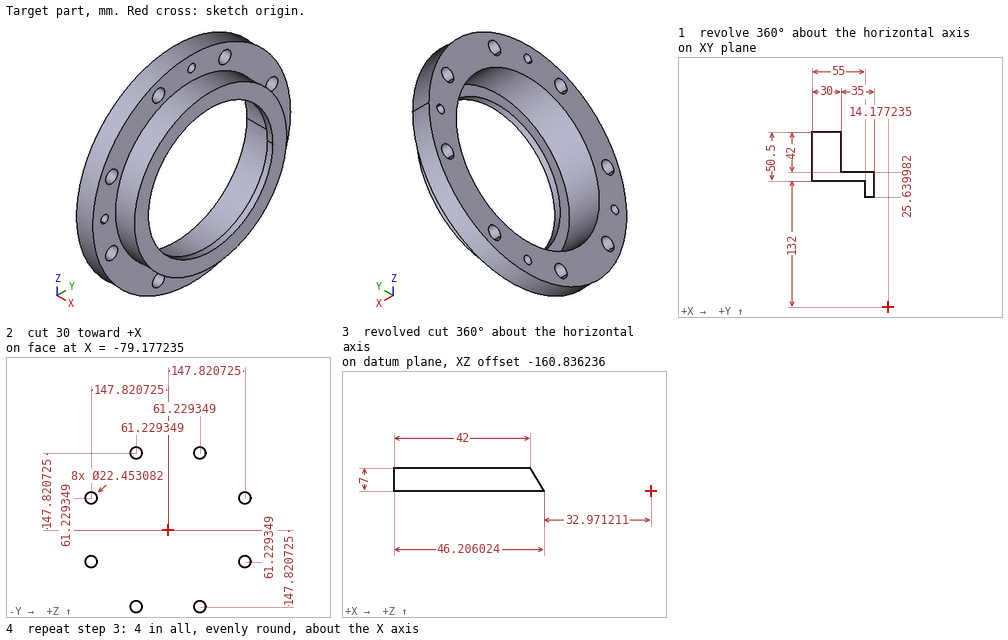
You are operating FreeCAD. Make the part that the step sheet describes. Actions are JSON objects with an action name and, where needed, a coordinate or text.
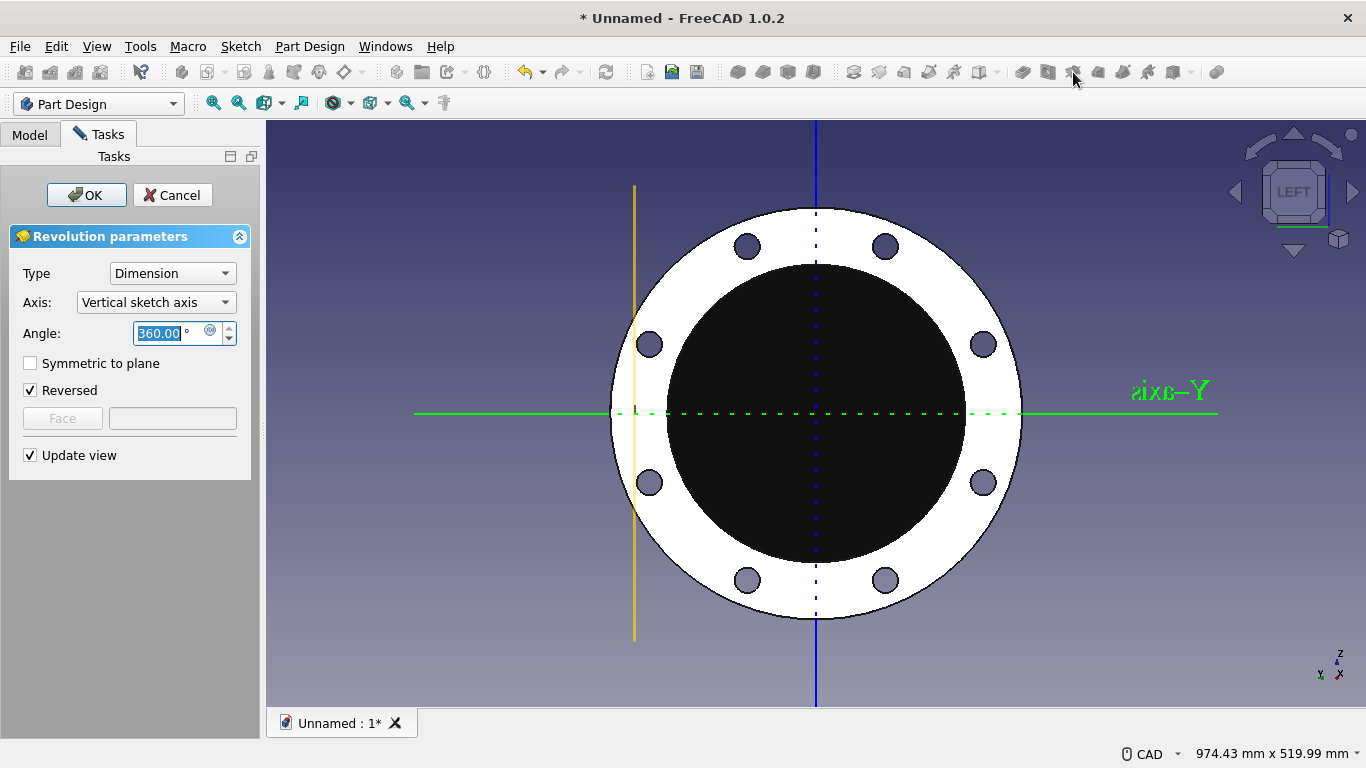
{"action": "left_click", "coordinate": [157, 302]}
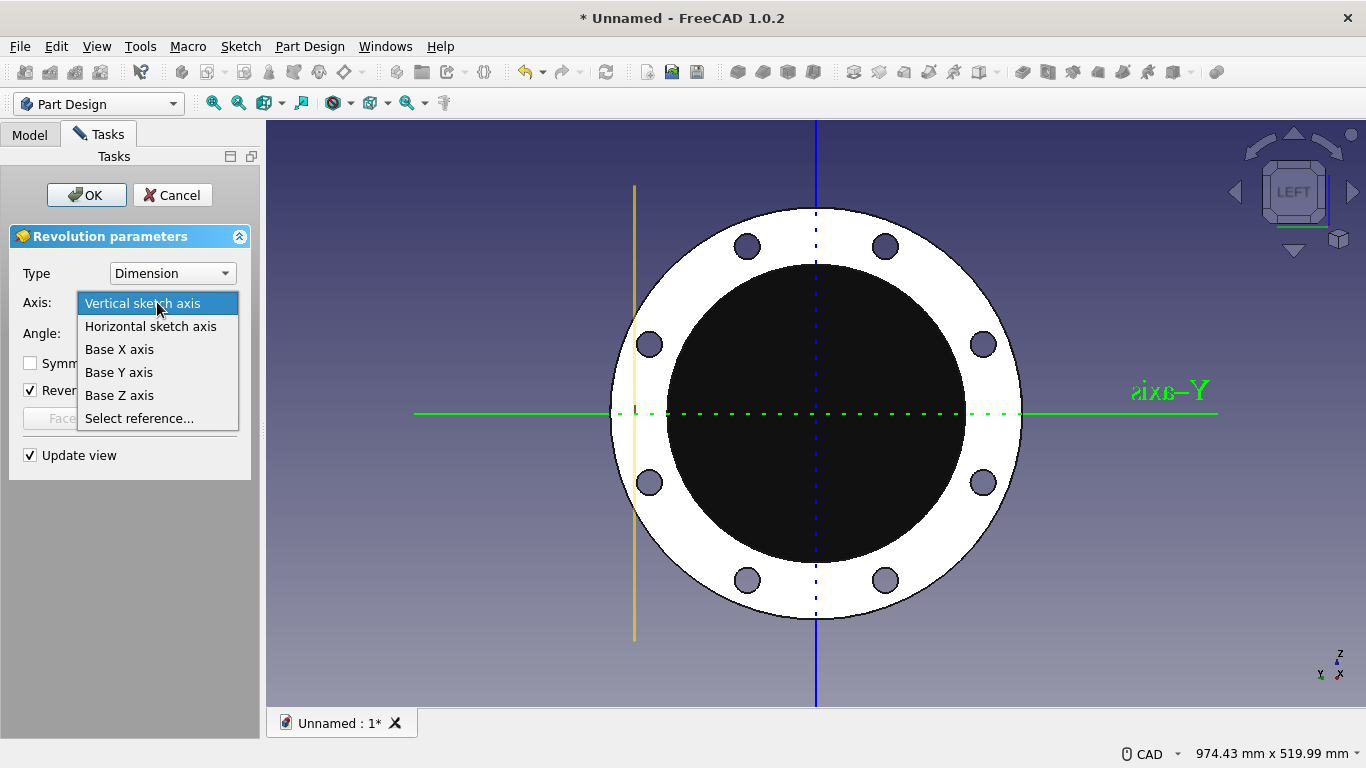
{"action": "left_click", "coordinate": [156, 326]}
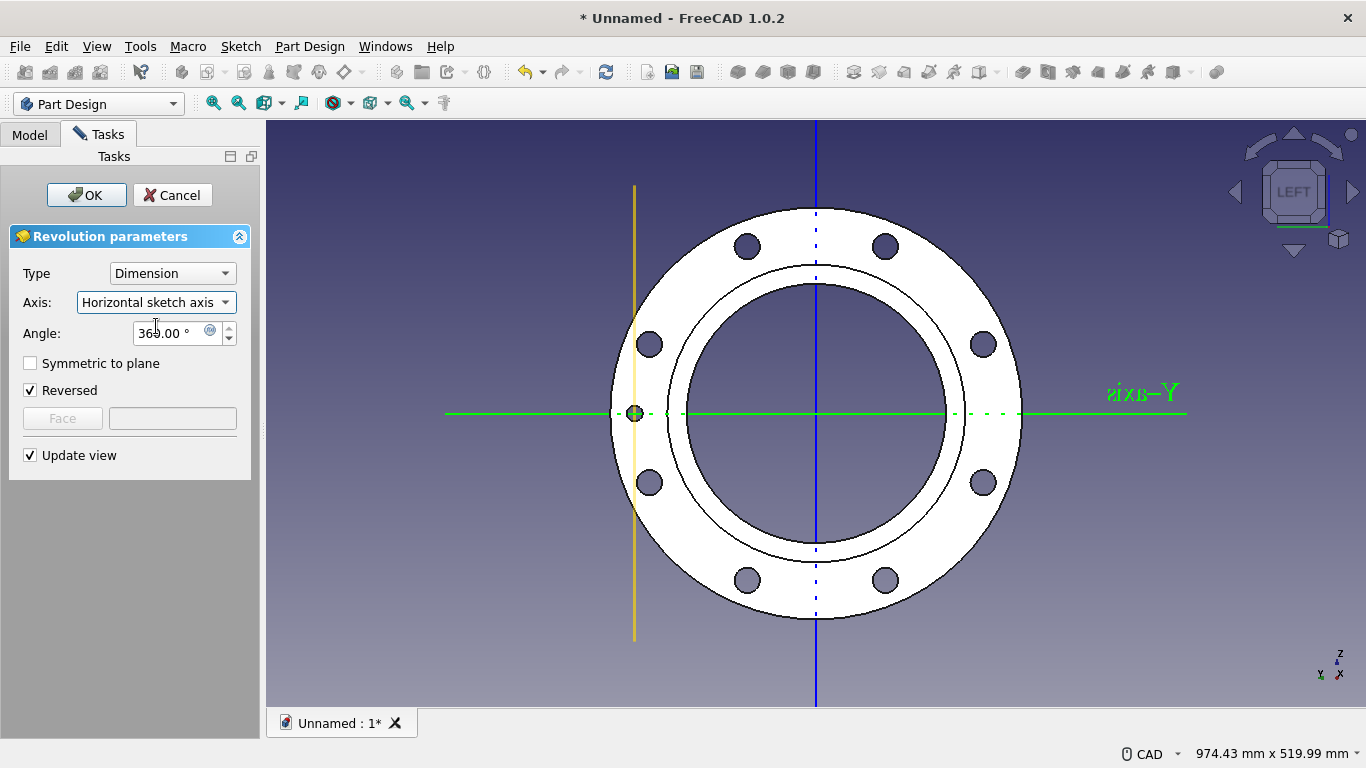
{"action": "left_click", "coordinate": [87, 195]}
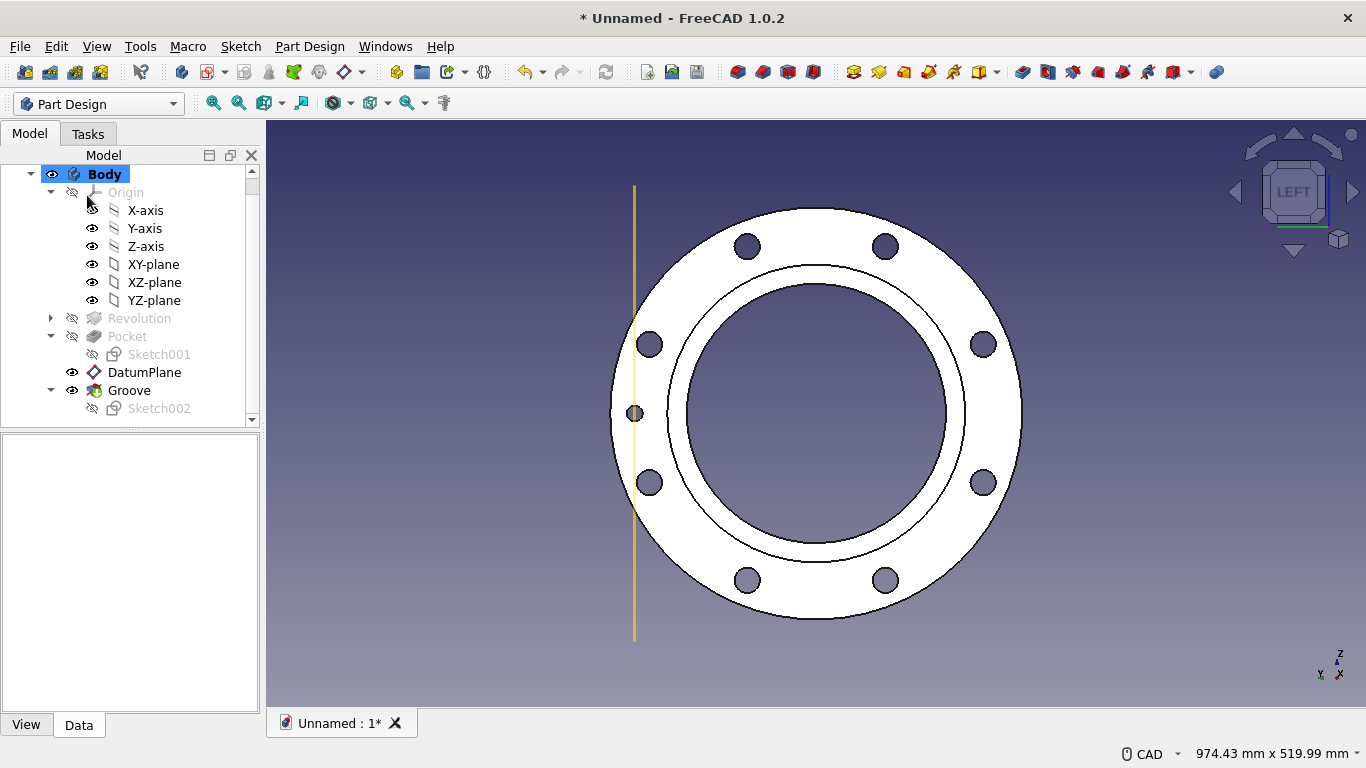
{"action": "left_click", "coordinate": [117, 372]}
{"action": "key", "text": "space"}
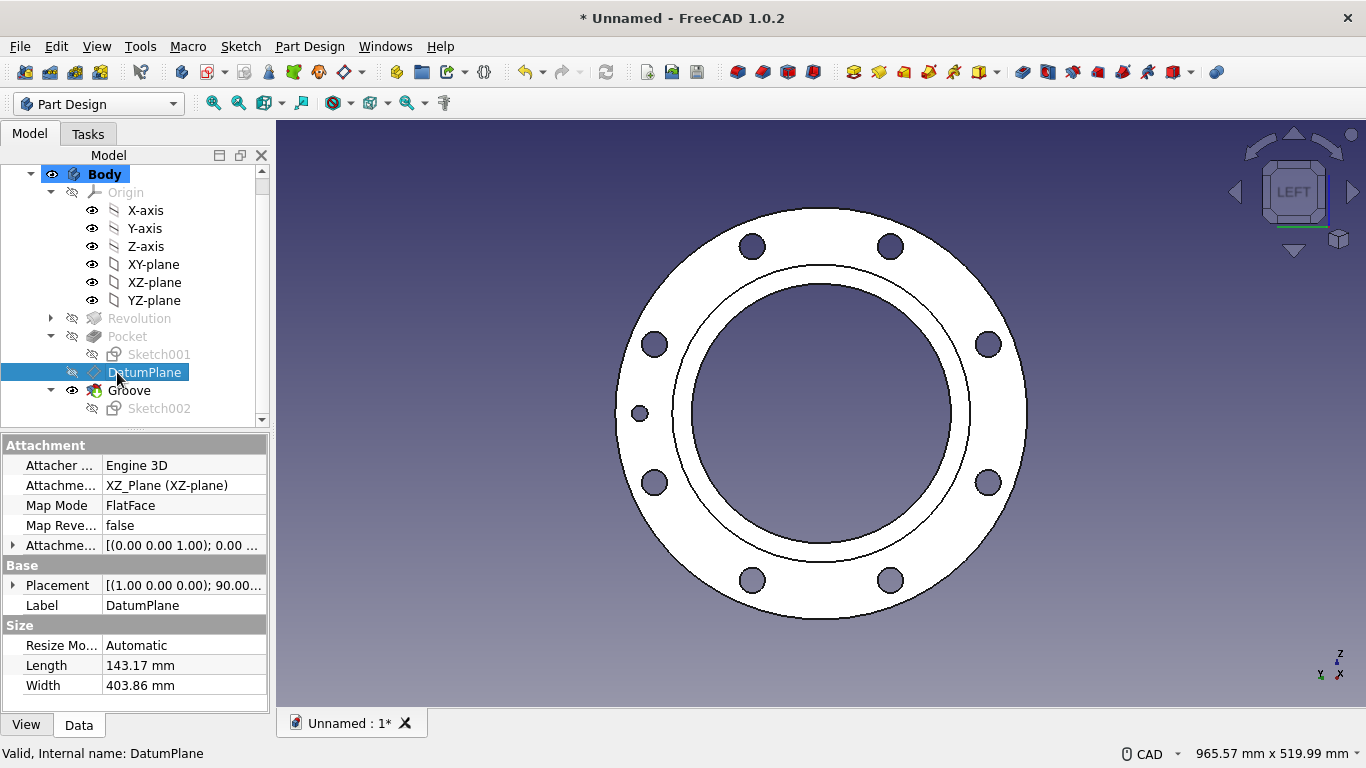
{"action": "left_click", "coordinate": [117, 390]}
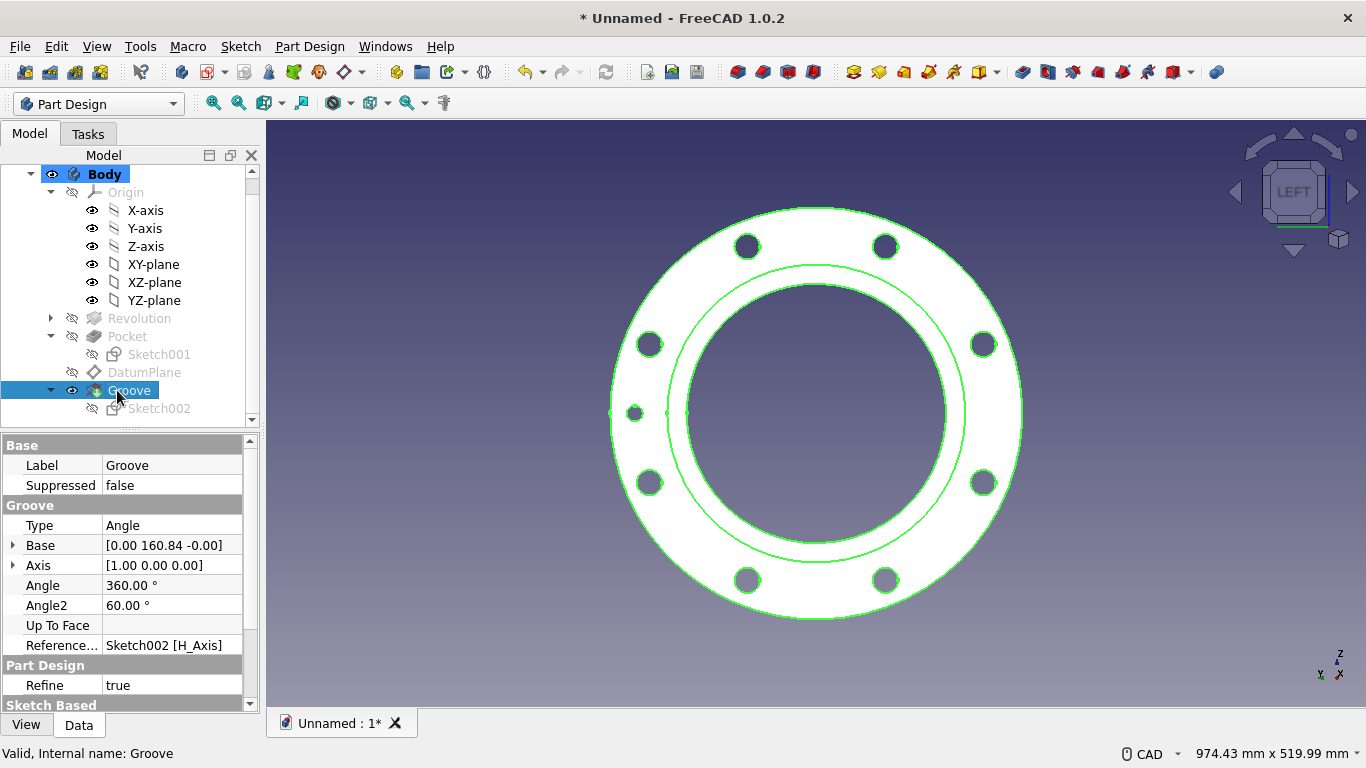
{"action": "left_click", "coordinate": [75, 72]}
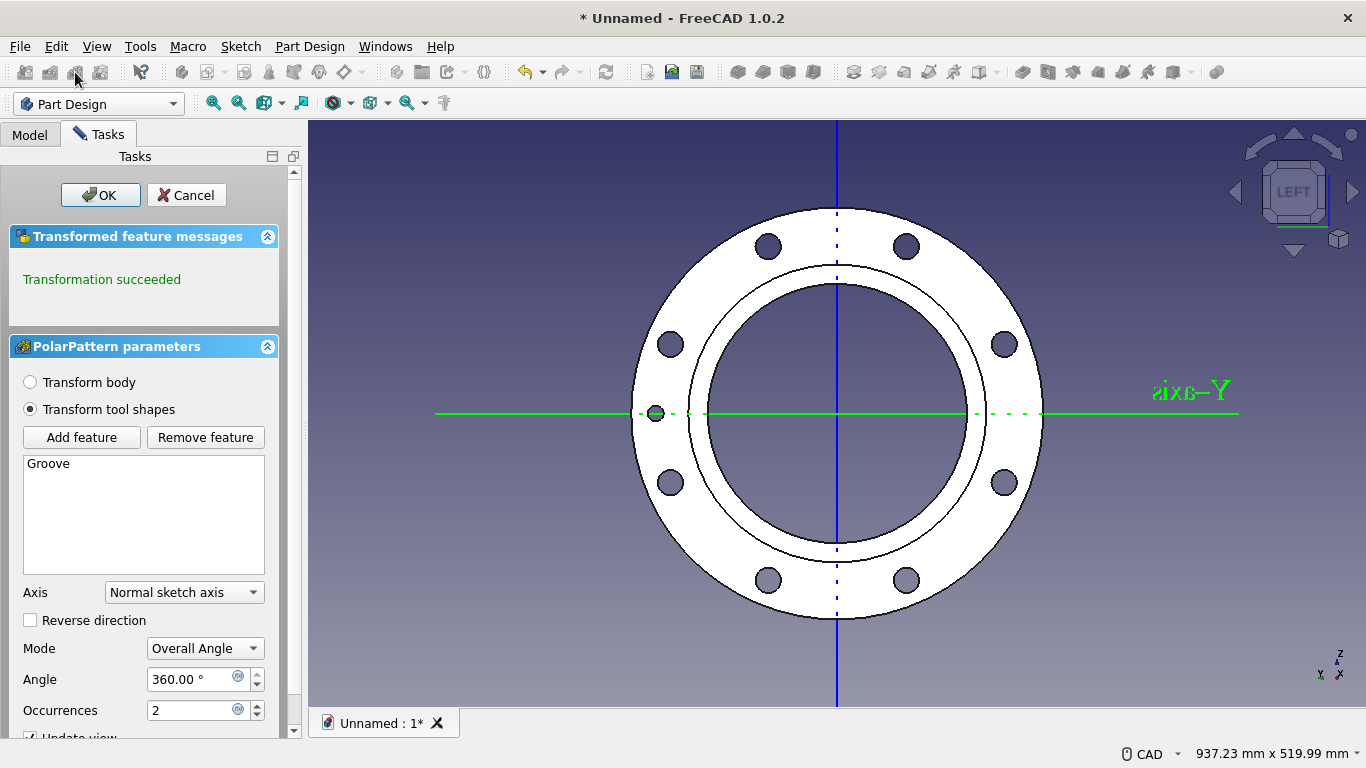
{"action": "left_click", "coordinate": [185, 592]}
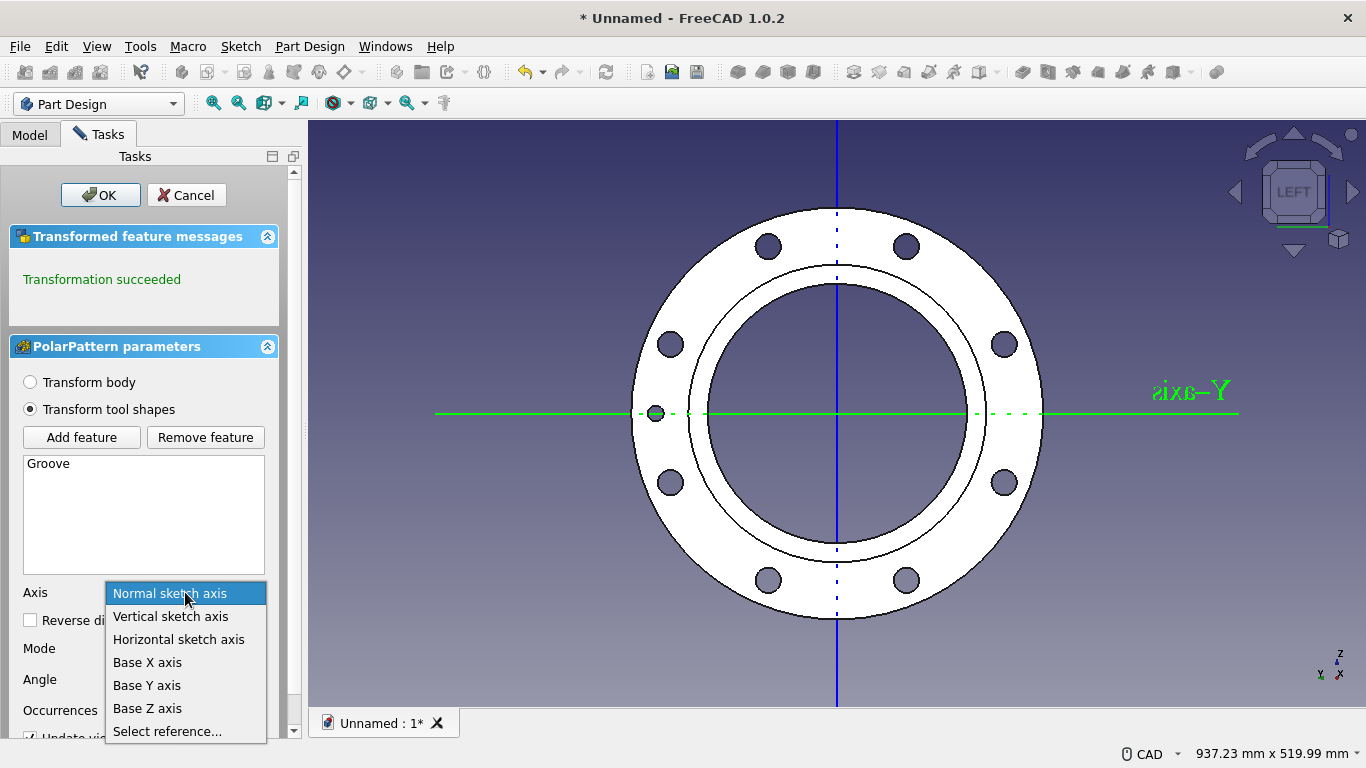
{"action": "left_click", "coordinate": [184, 662]}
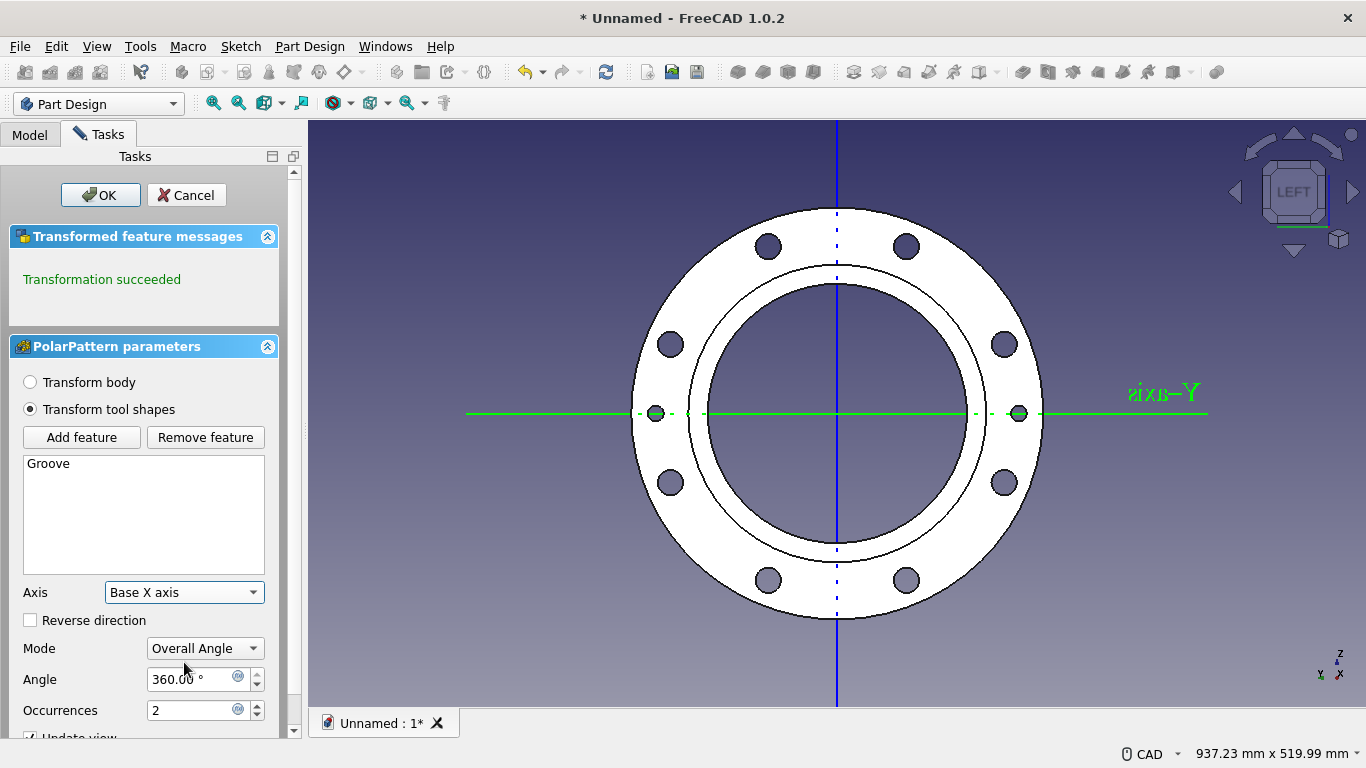
{"action": "triple_click", "coordinate": [199, 710]}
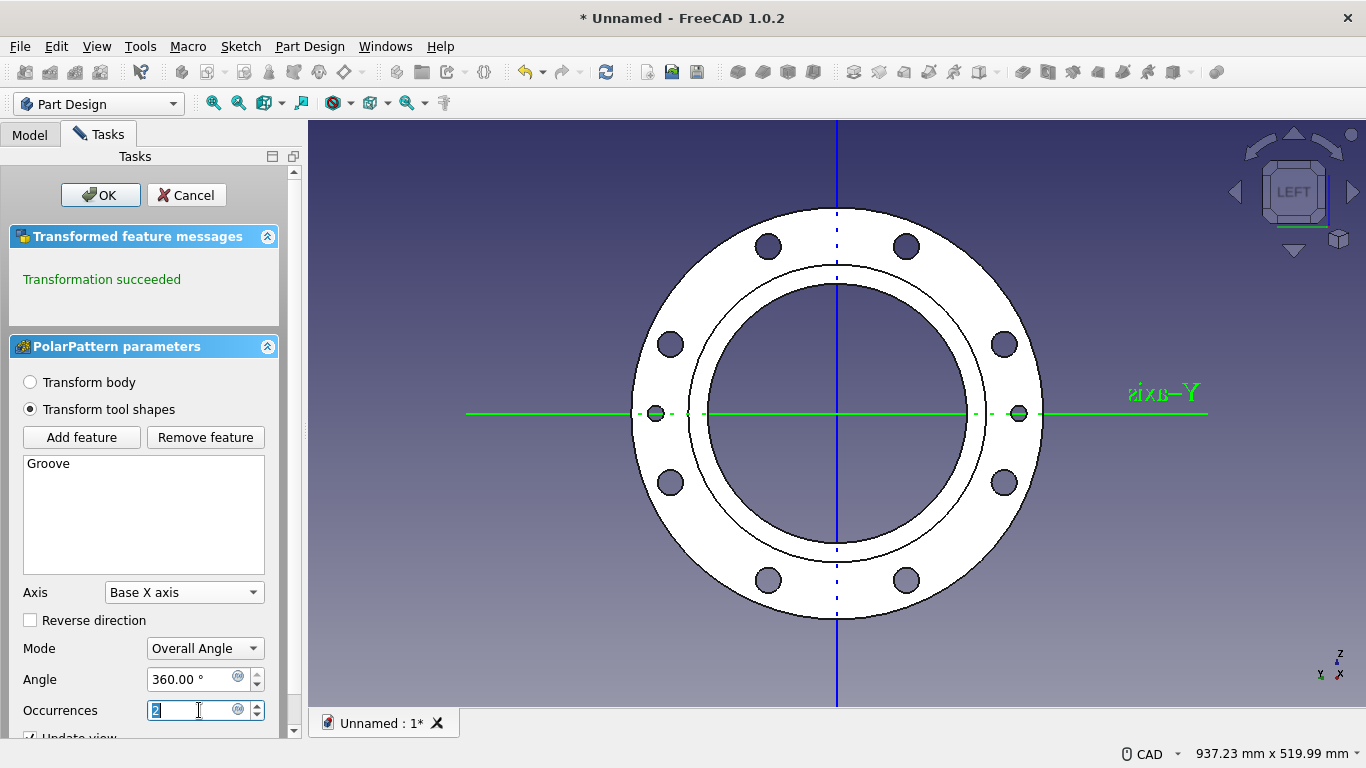
{"action": "type", "text": "4"}
{"action": "key", "text": "Tab"}